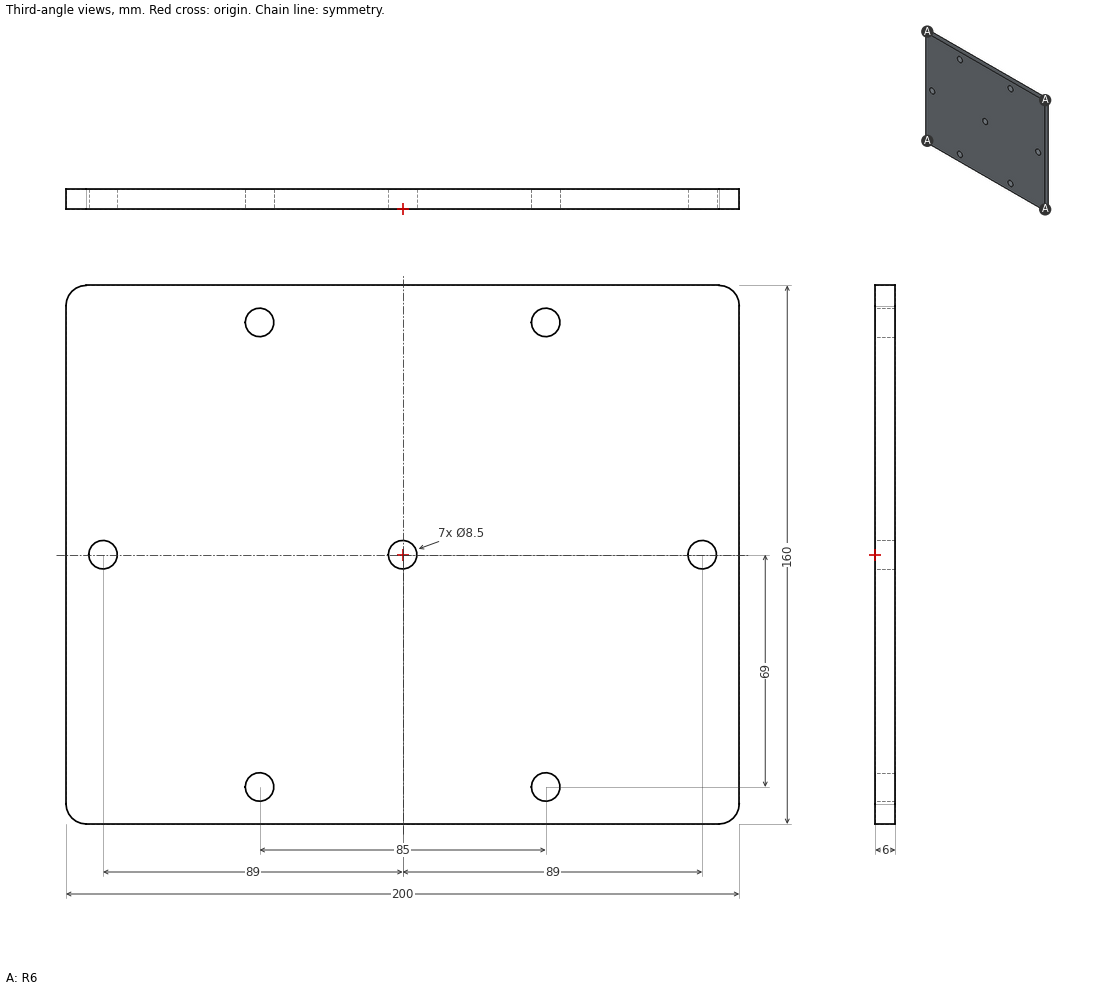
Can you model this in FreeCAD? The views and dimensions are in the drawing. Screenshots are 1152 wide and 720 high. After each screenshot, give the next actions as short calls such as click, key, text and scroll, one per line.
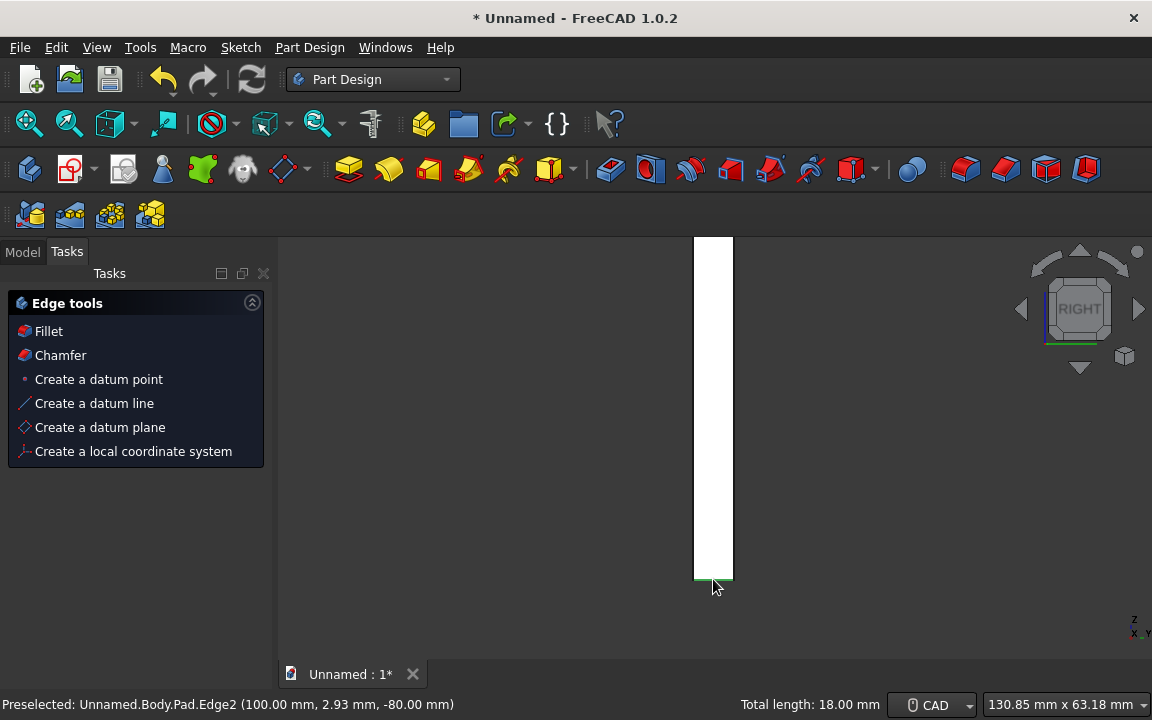
click(30, 124)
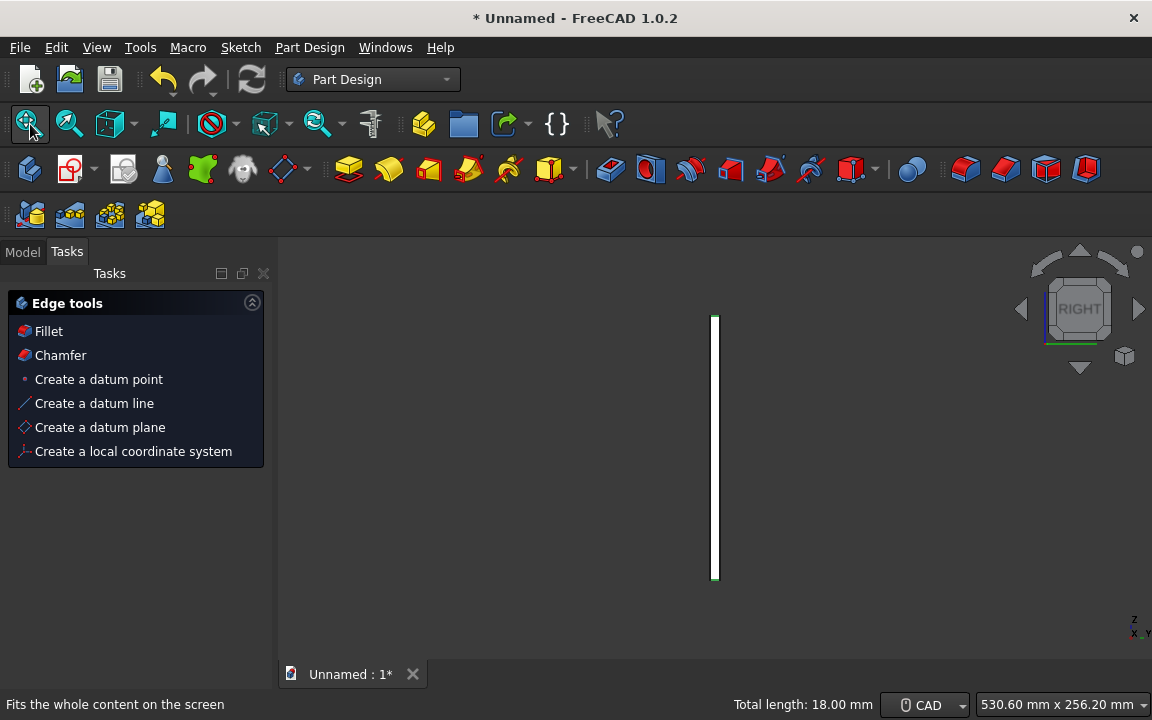
key(5)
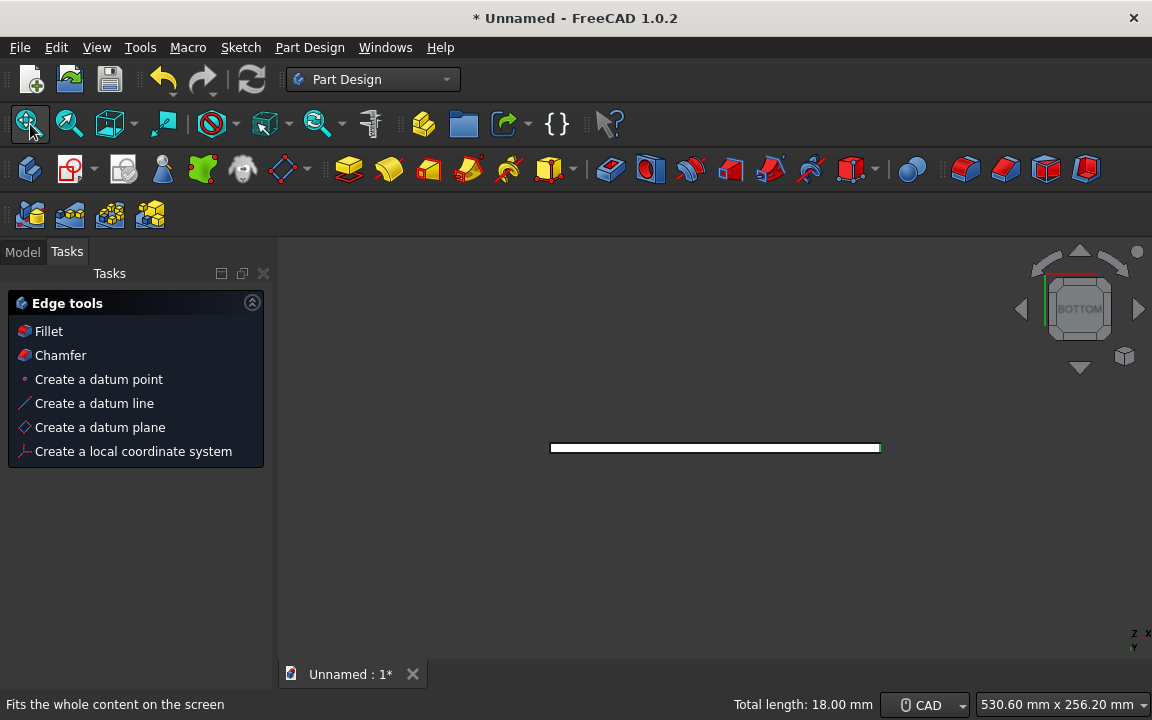
click(30, 124)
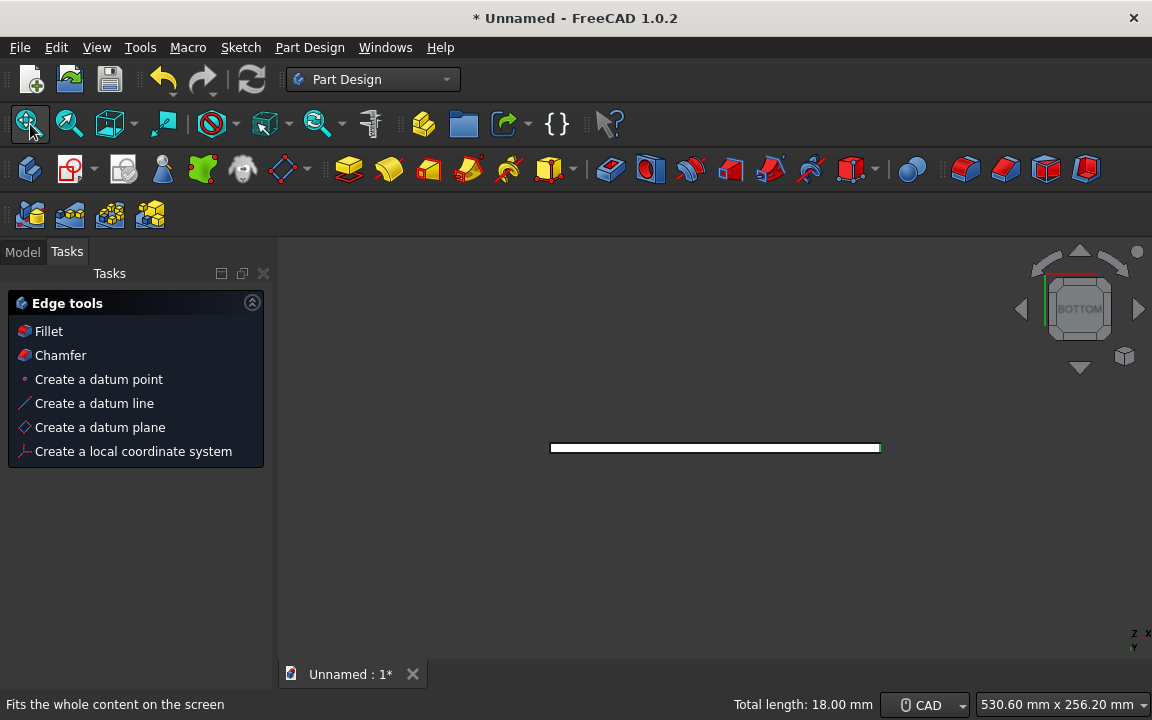
click(550, 449, ctrl)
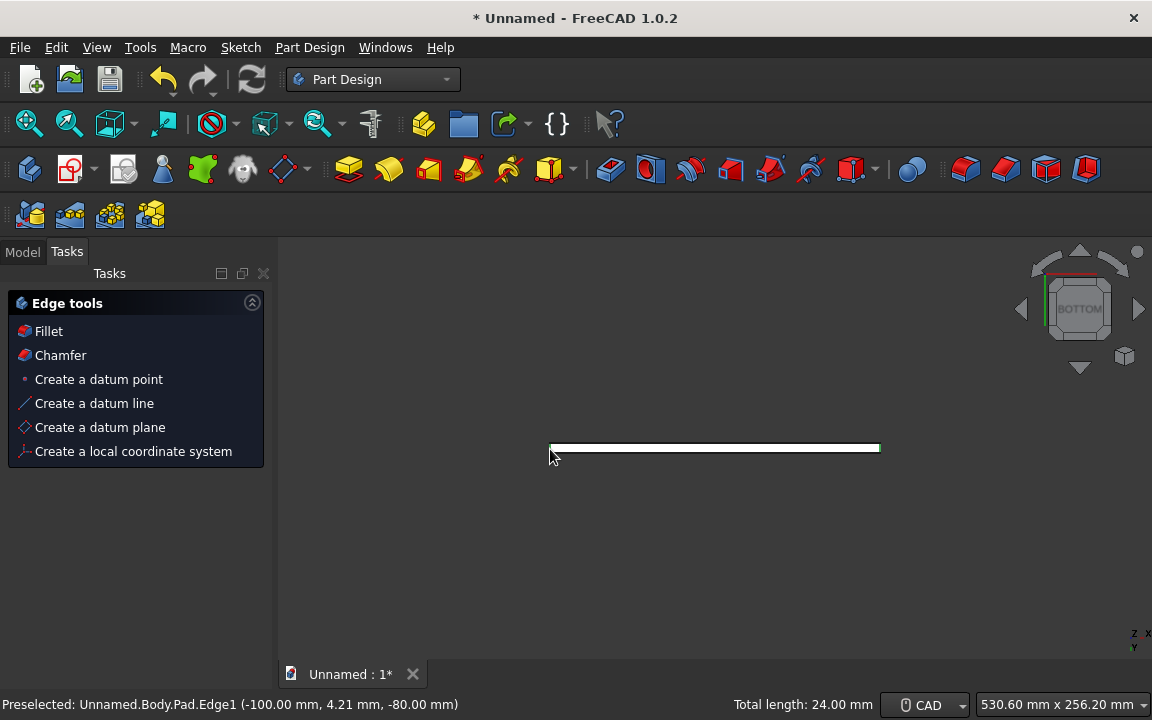
click(966, 170)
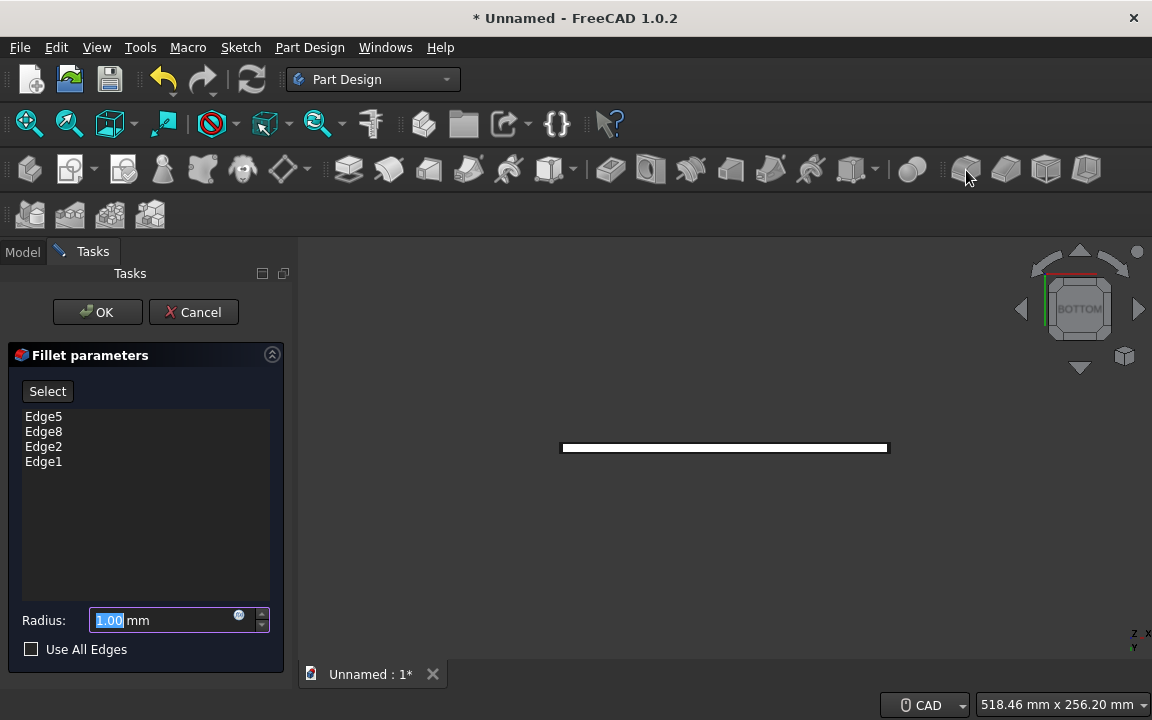
text(6)
key(Tab)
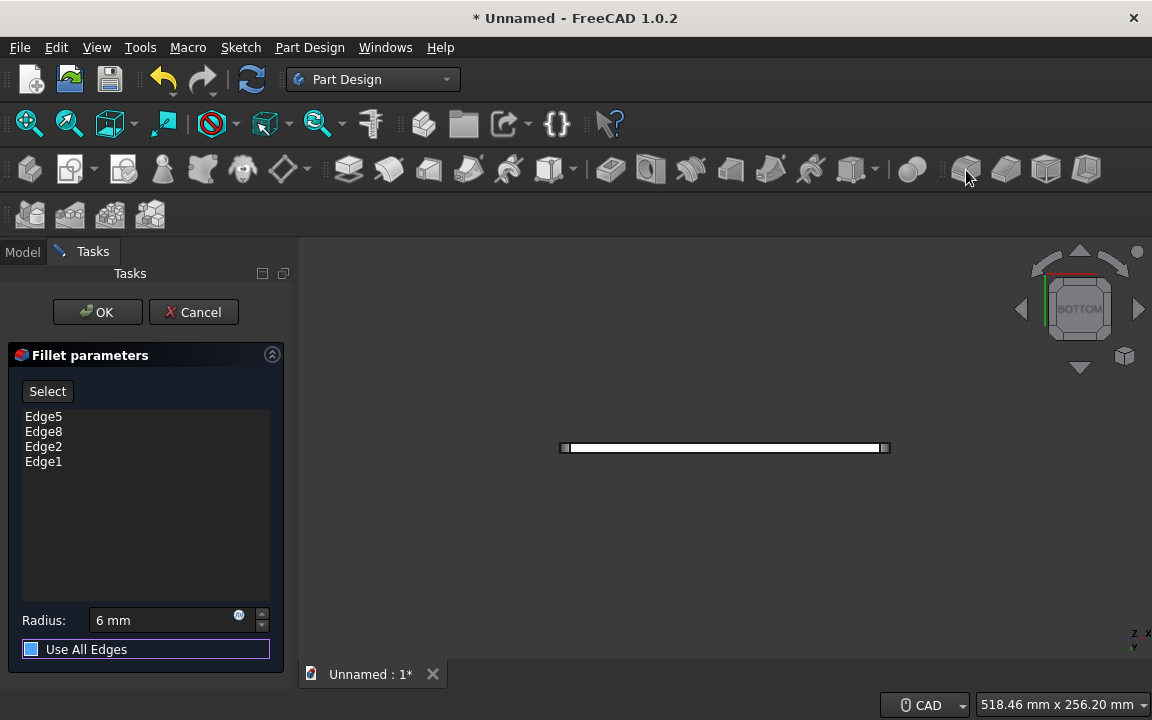
click(98, 312)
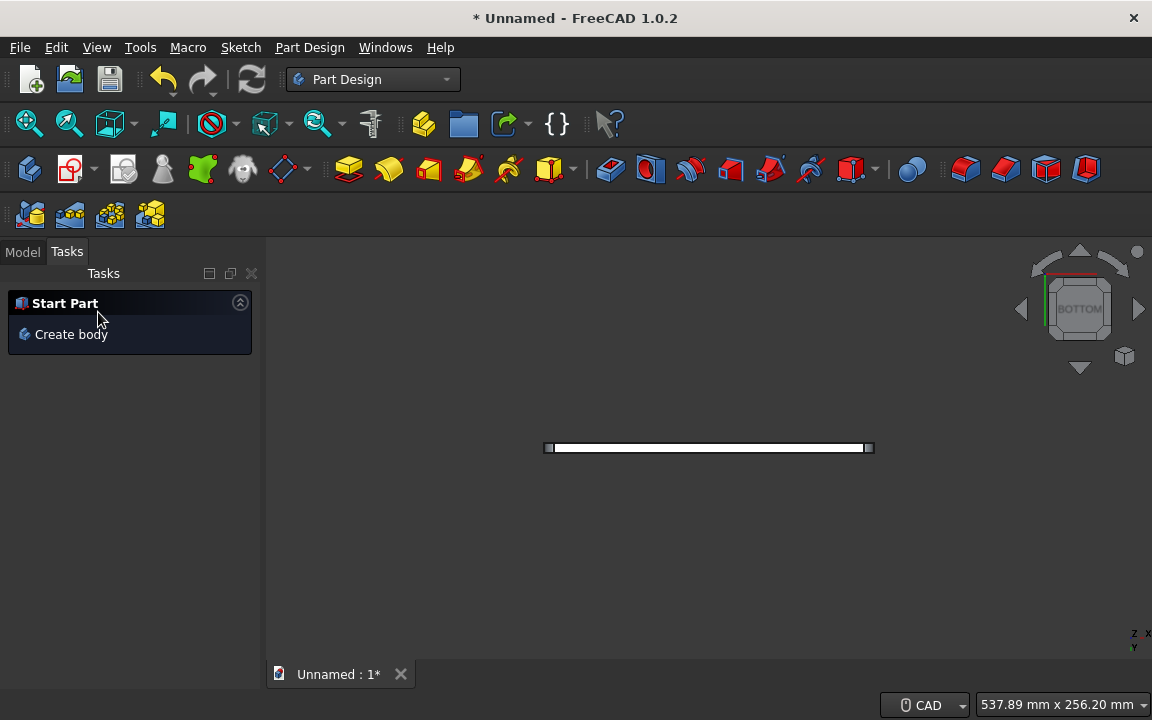
click(30, 124)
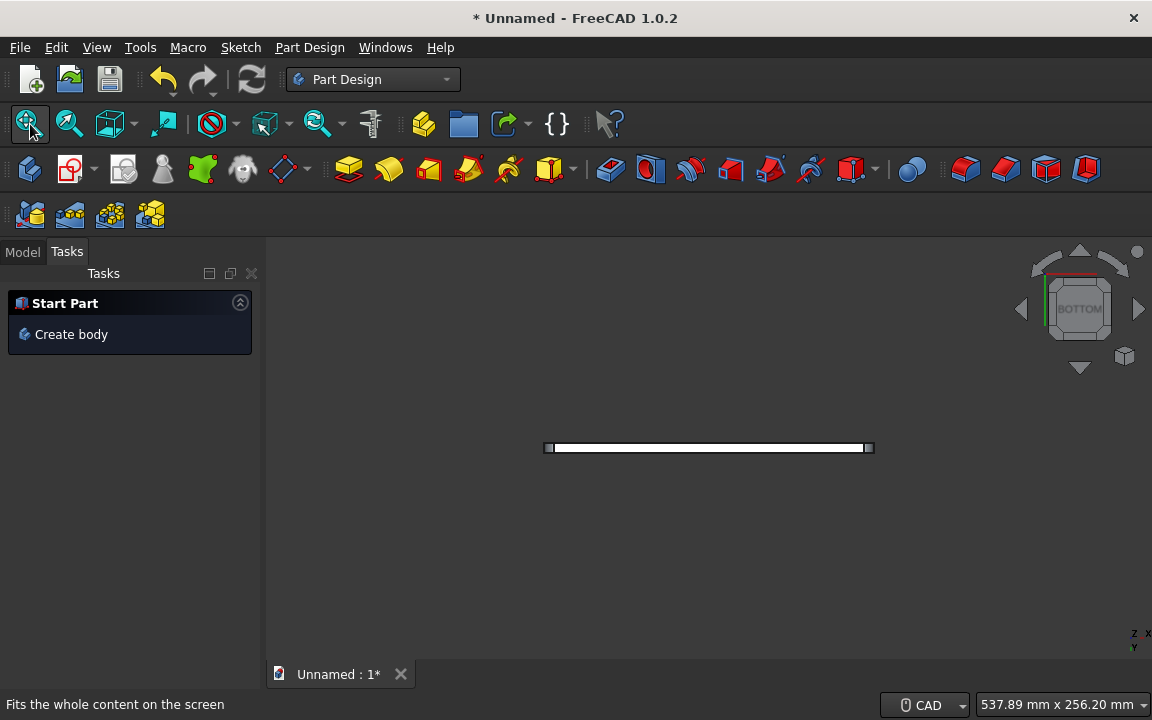
key(4)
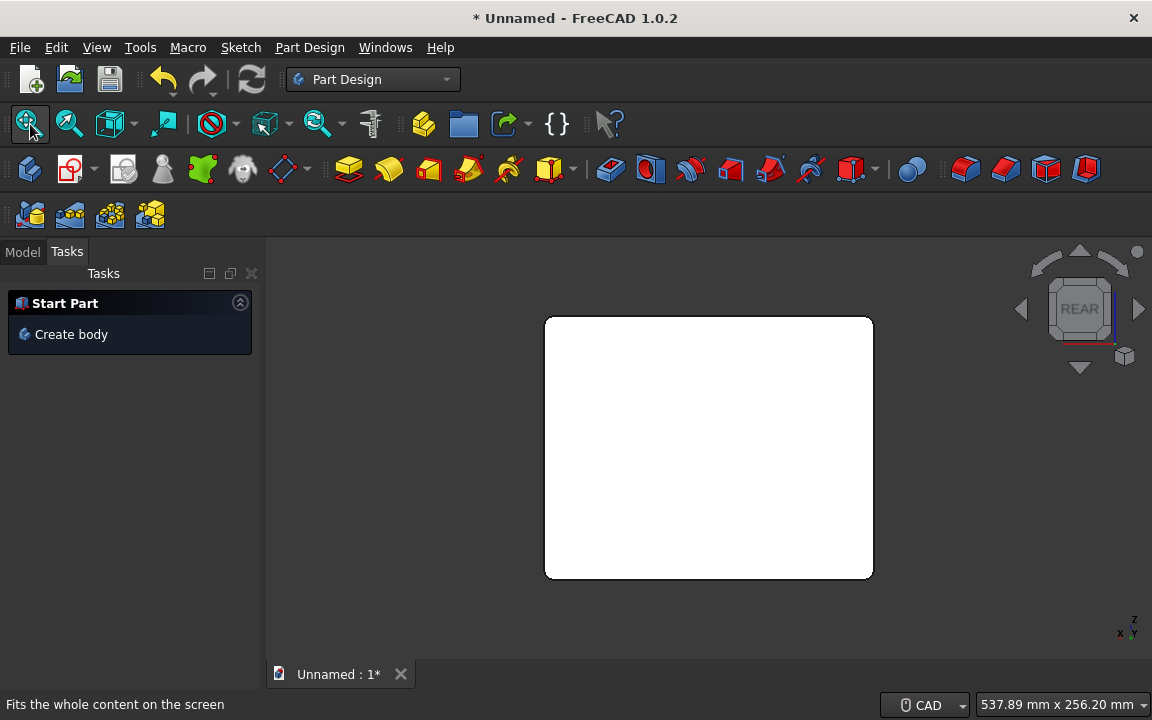
click(709, 447)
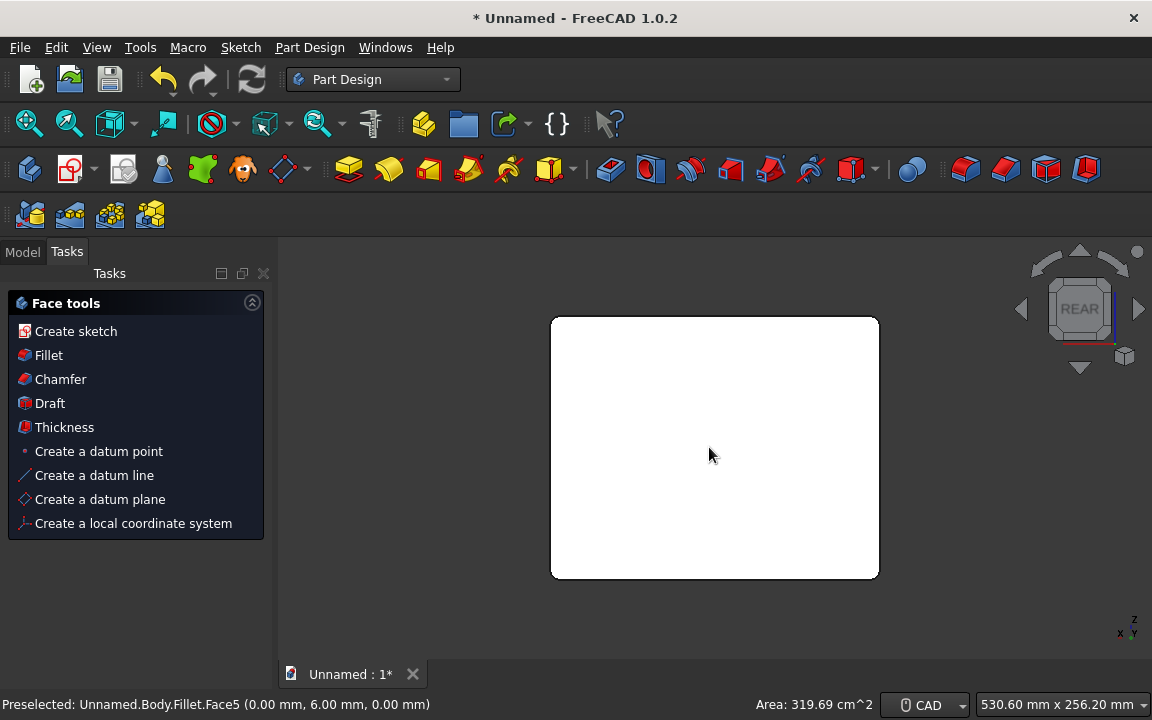
click(70, 170)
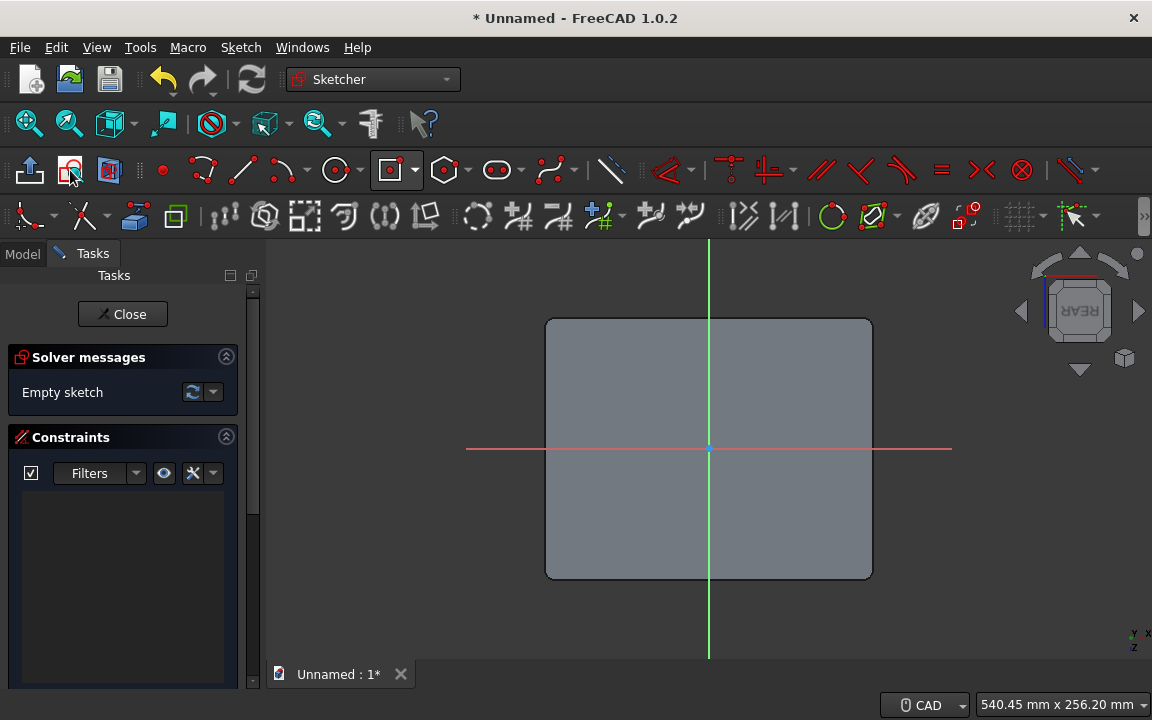
click(336, 170)